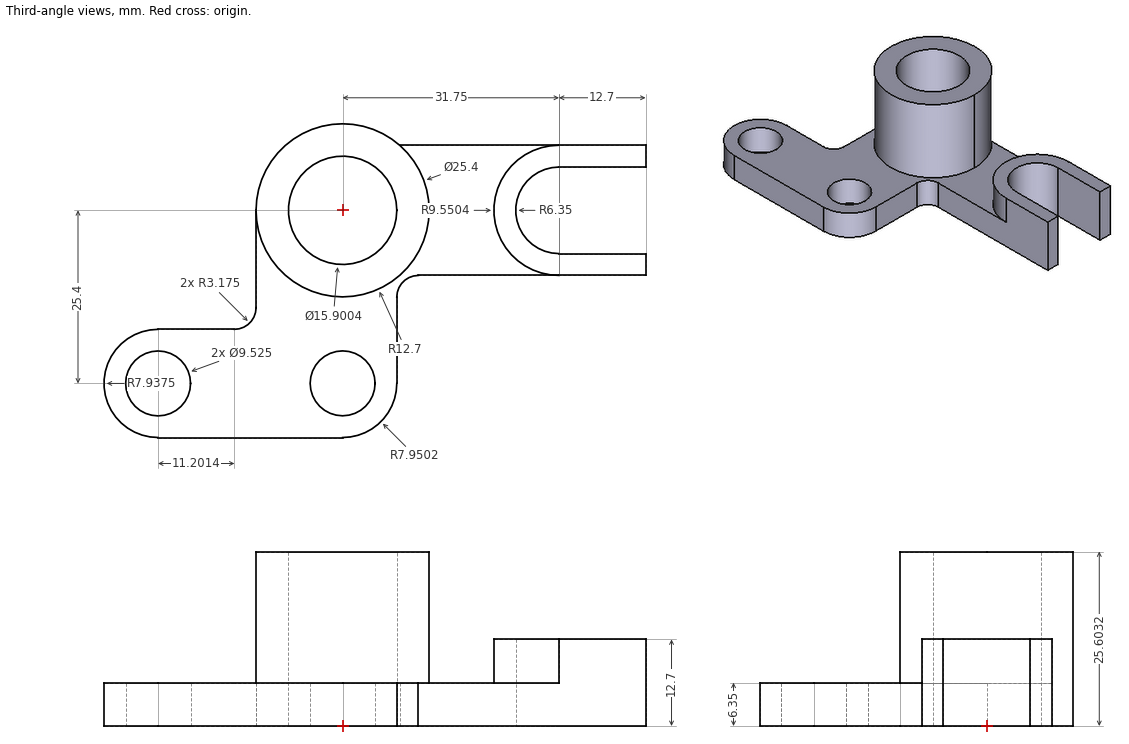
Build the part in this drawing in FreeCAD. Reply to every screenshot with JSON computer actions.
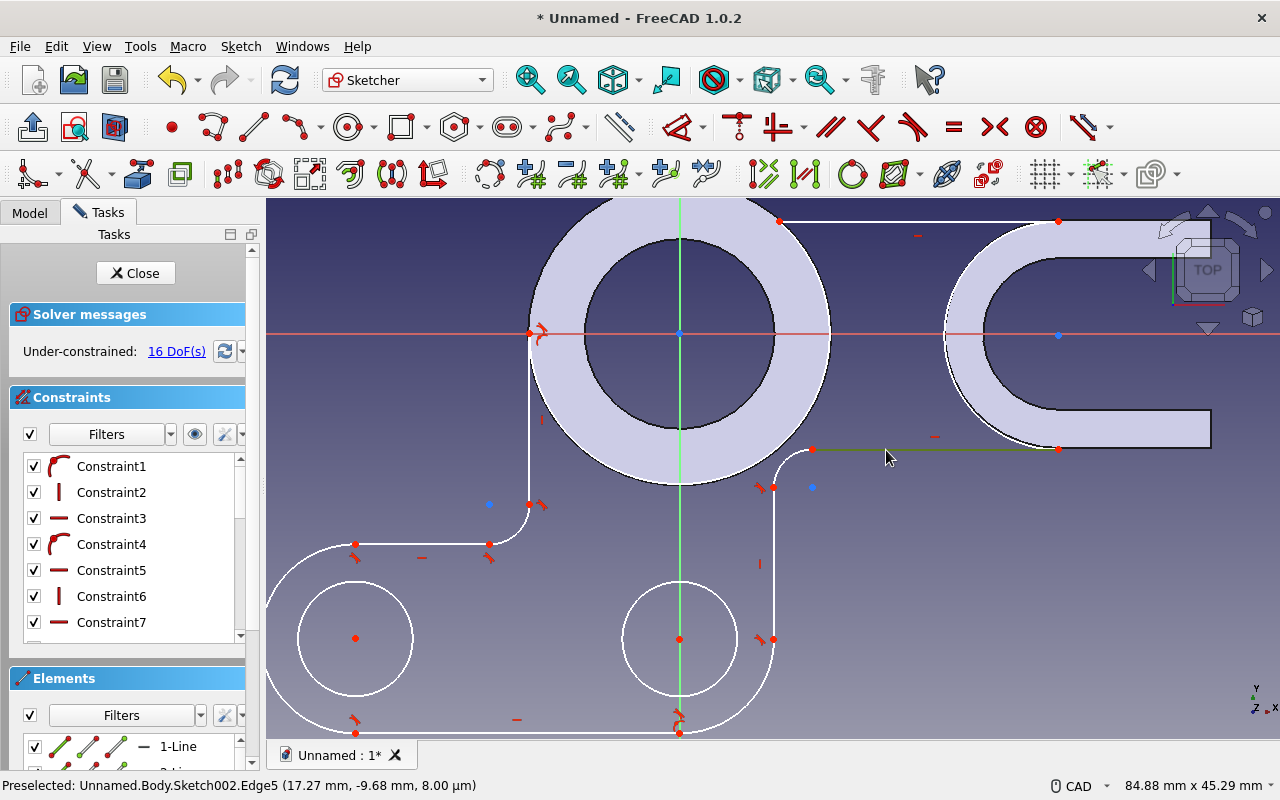
{"action": "left_click", "coordinate": [795, 454]}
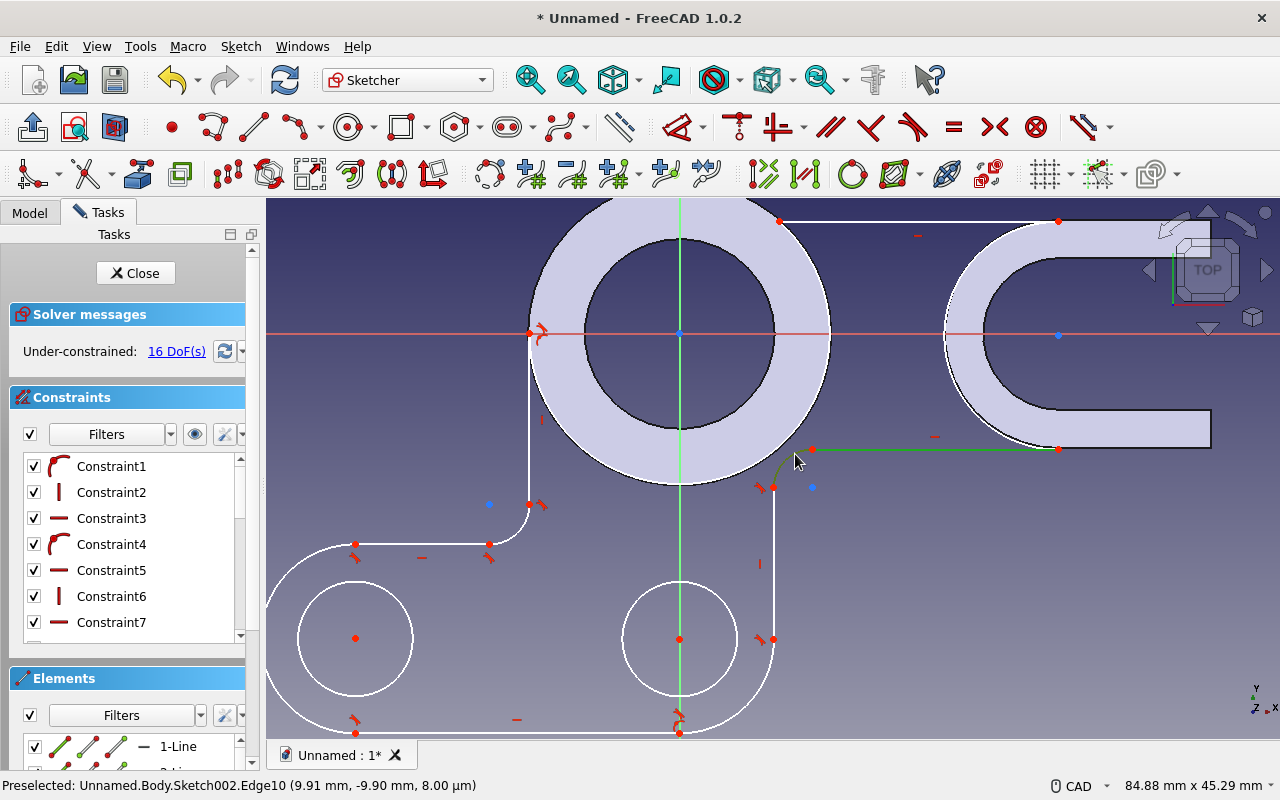
{"action": "left_click", "coordinate": [913, 128]}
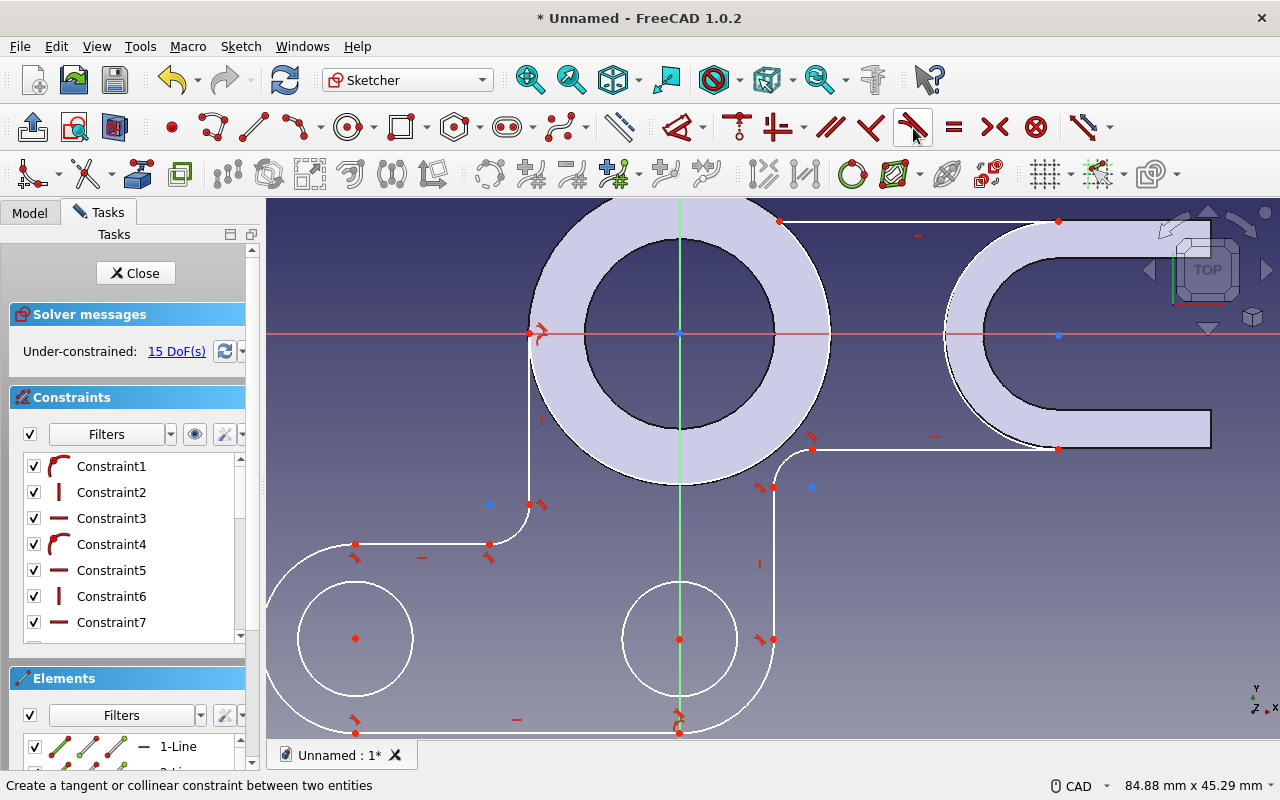
{"action": "left_click", "coordinate": [886, 450]}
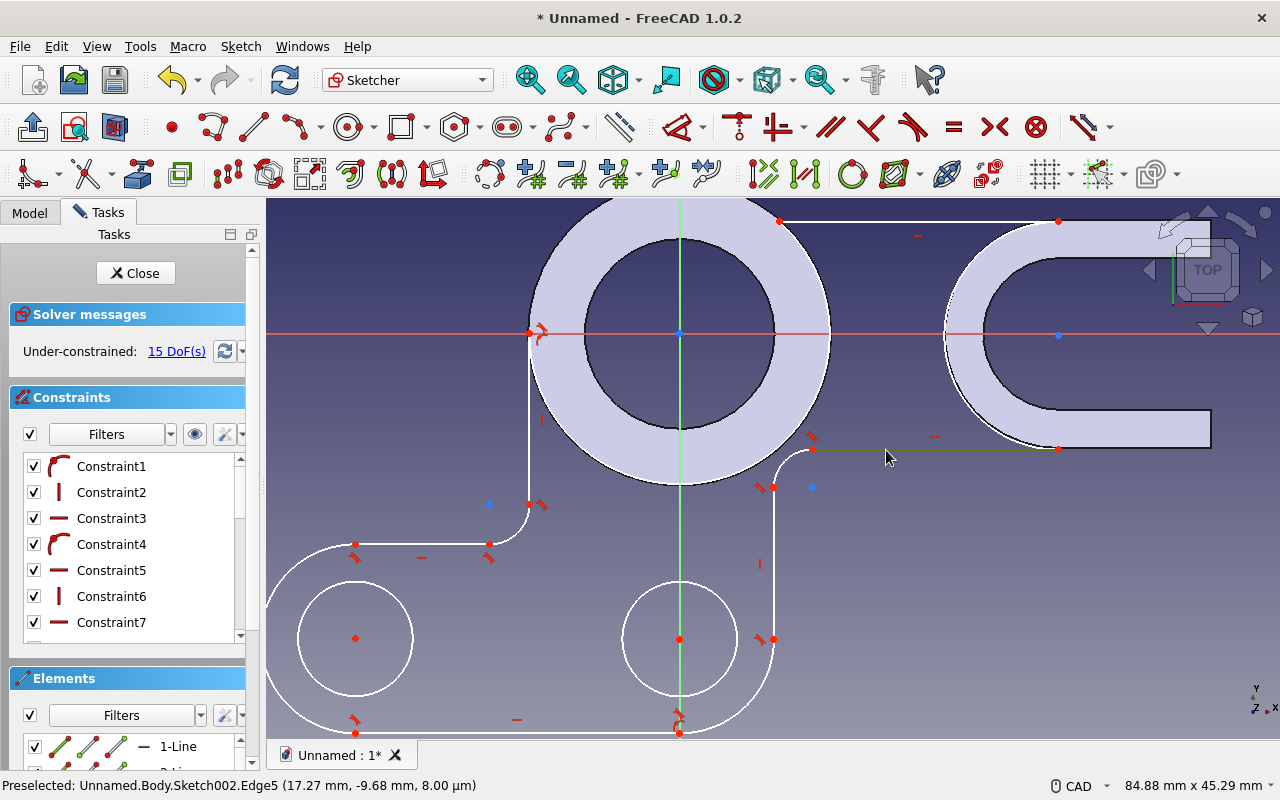
{"action": "left_click", "coordinate": [966, 269]}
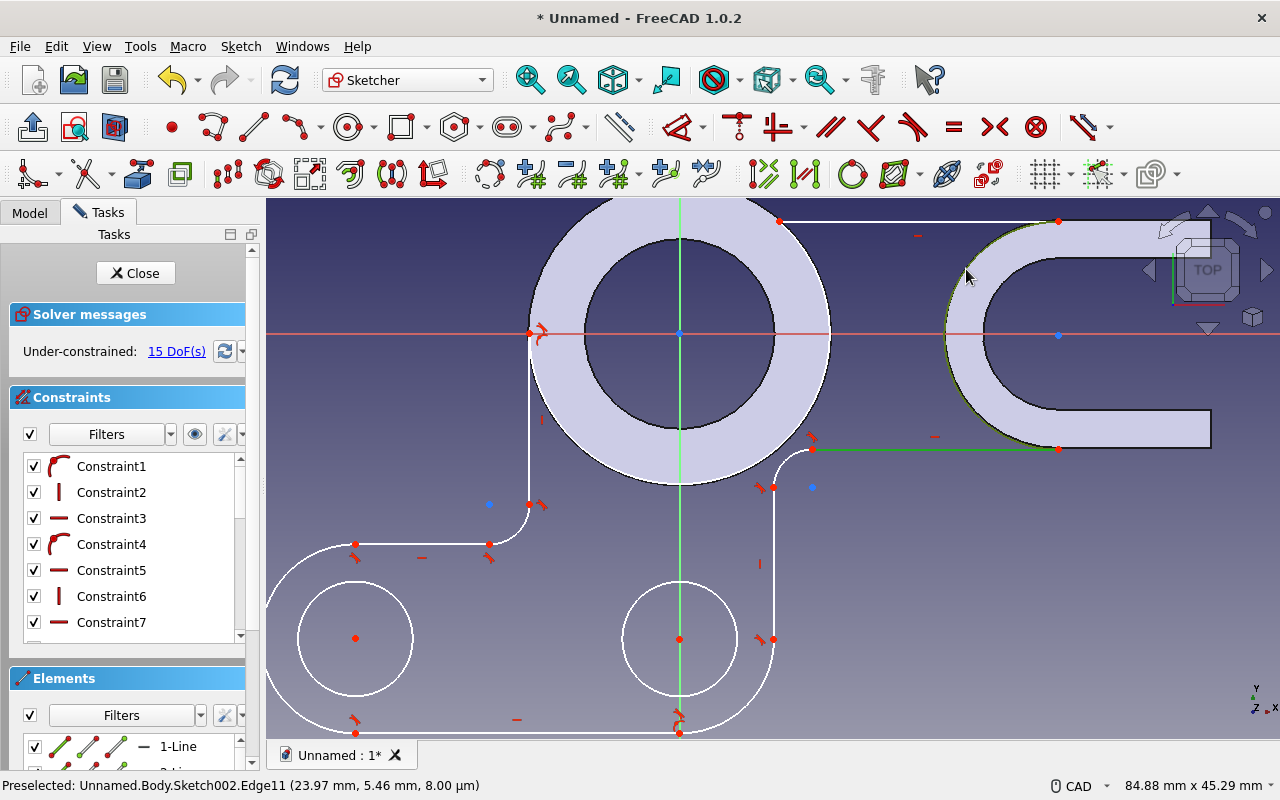
{"action": "key", "text": "t"}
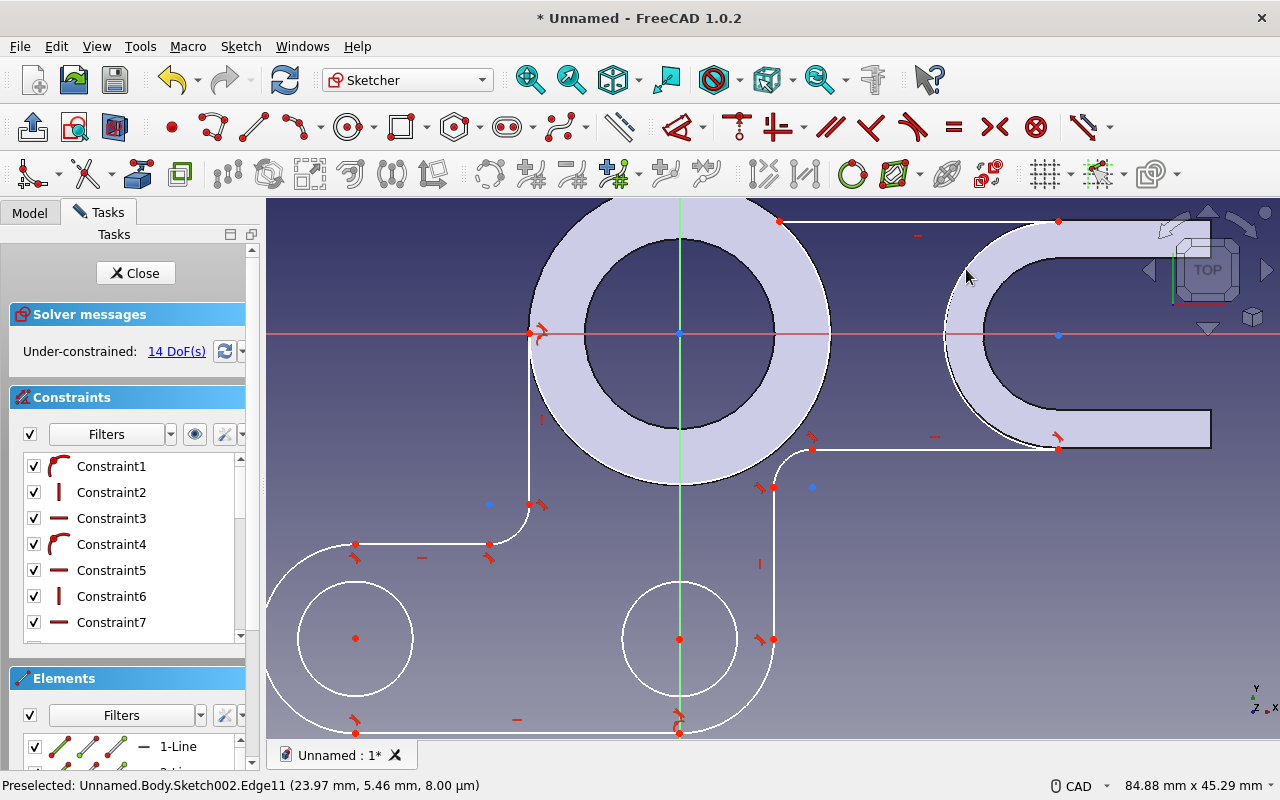
{"action": "scroll", "coordinate": [795, 453], "scroll_direction": "down", "scroll_amount": 2}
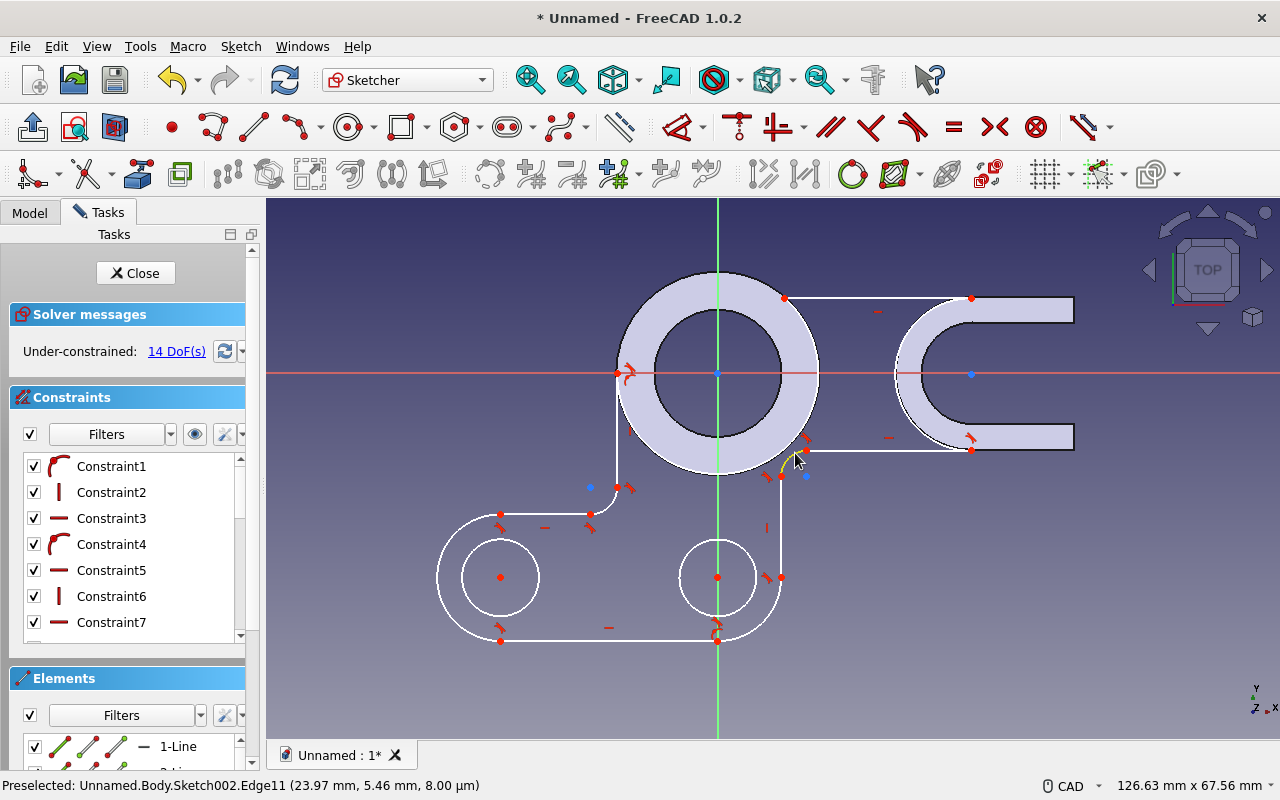
{"action": "left_click", "coordinate": [916, 298]}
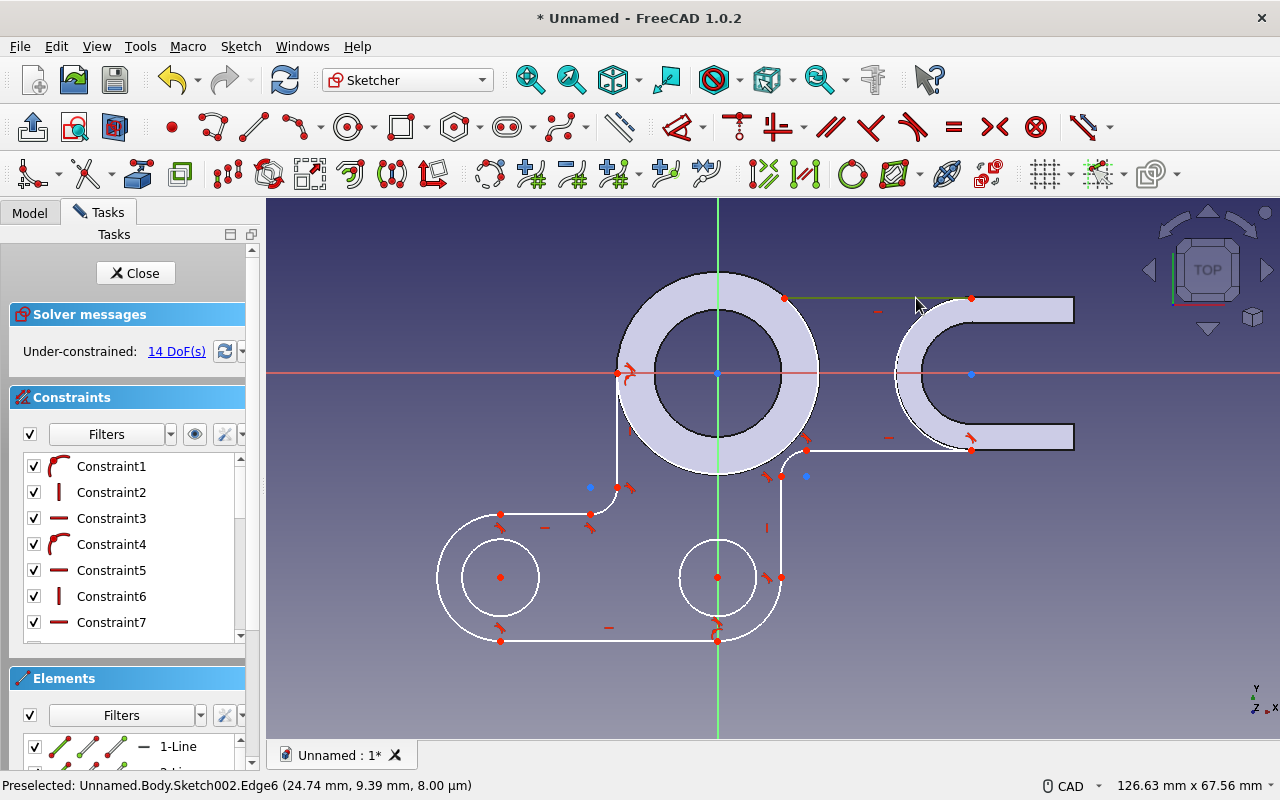
{"action": "left_click", "coordinate": [910, 330]}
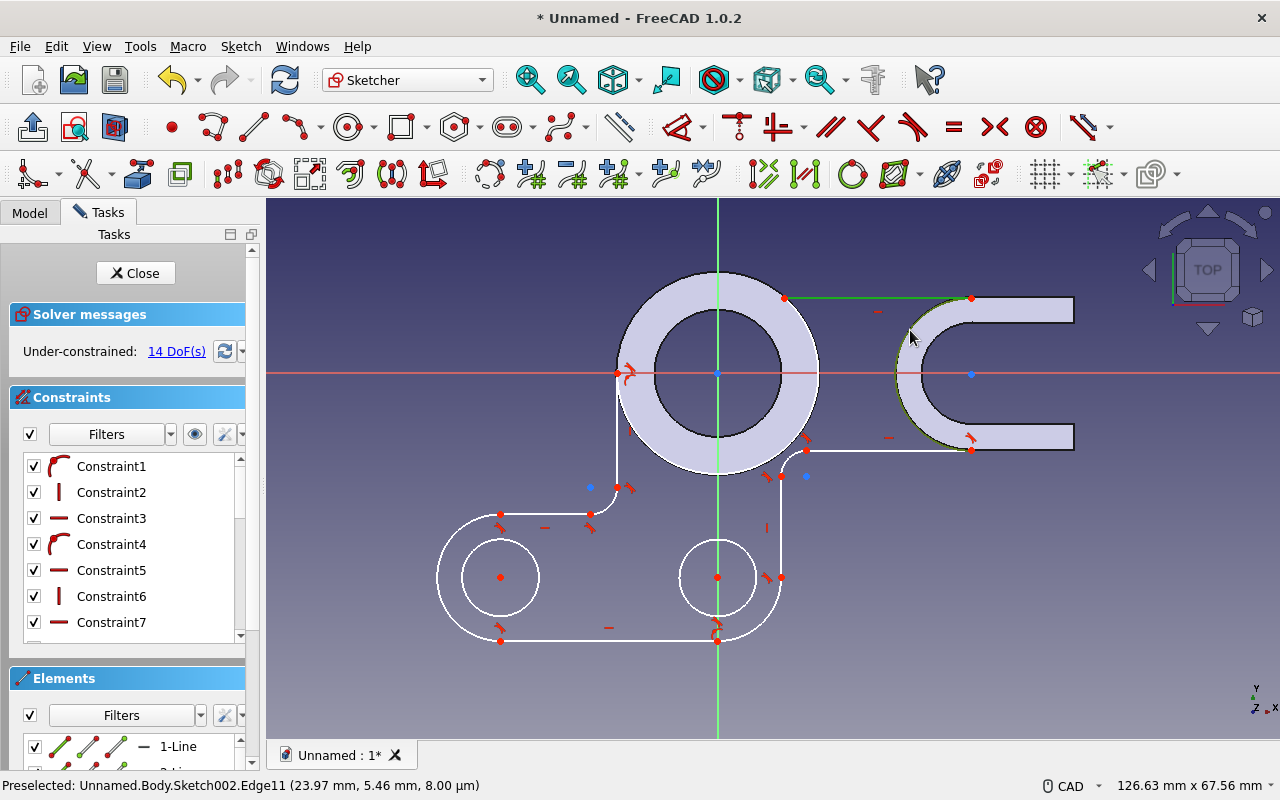
{"action": "key", "text": "t"}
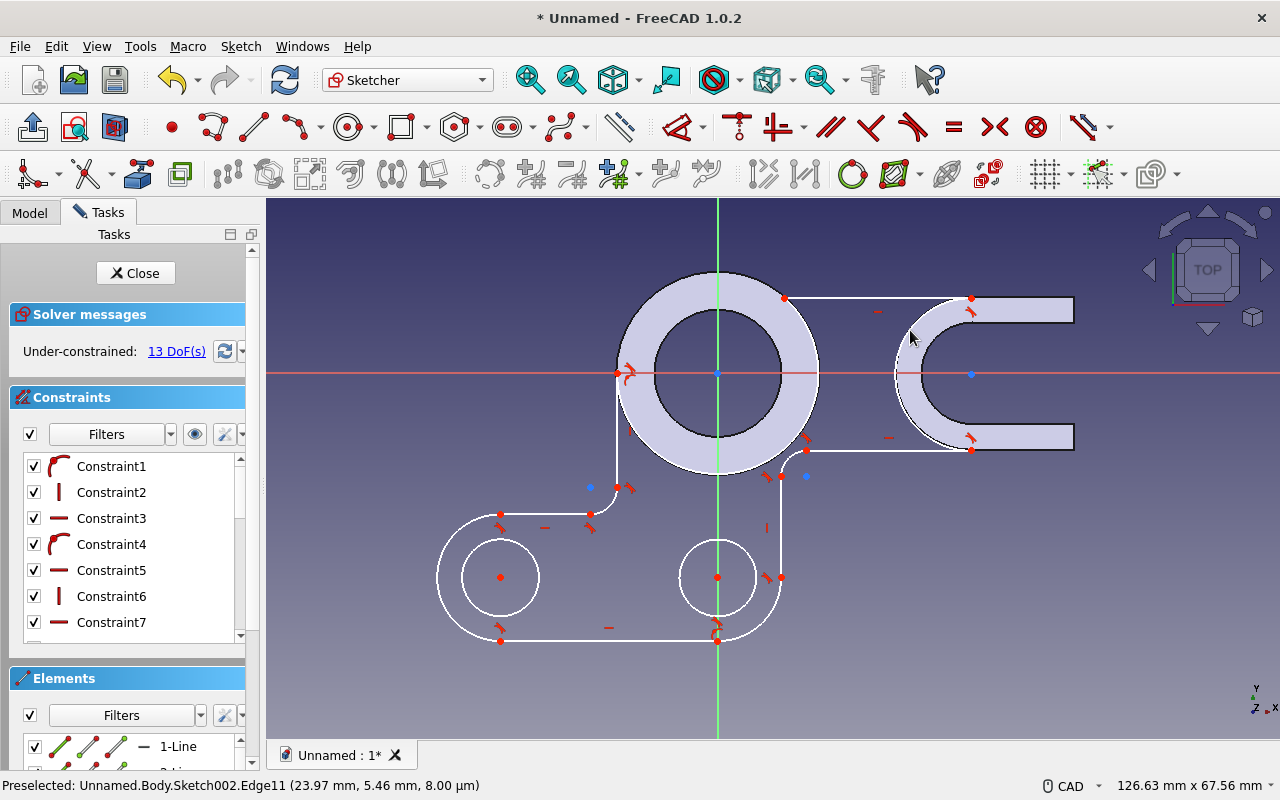
{"action": "left_click", "coordinate": [603, 511]}